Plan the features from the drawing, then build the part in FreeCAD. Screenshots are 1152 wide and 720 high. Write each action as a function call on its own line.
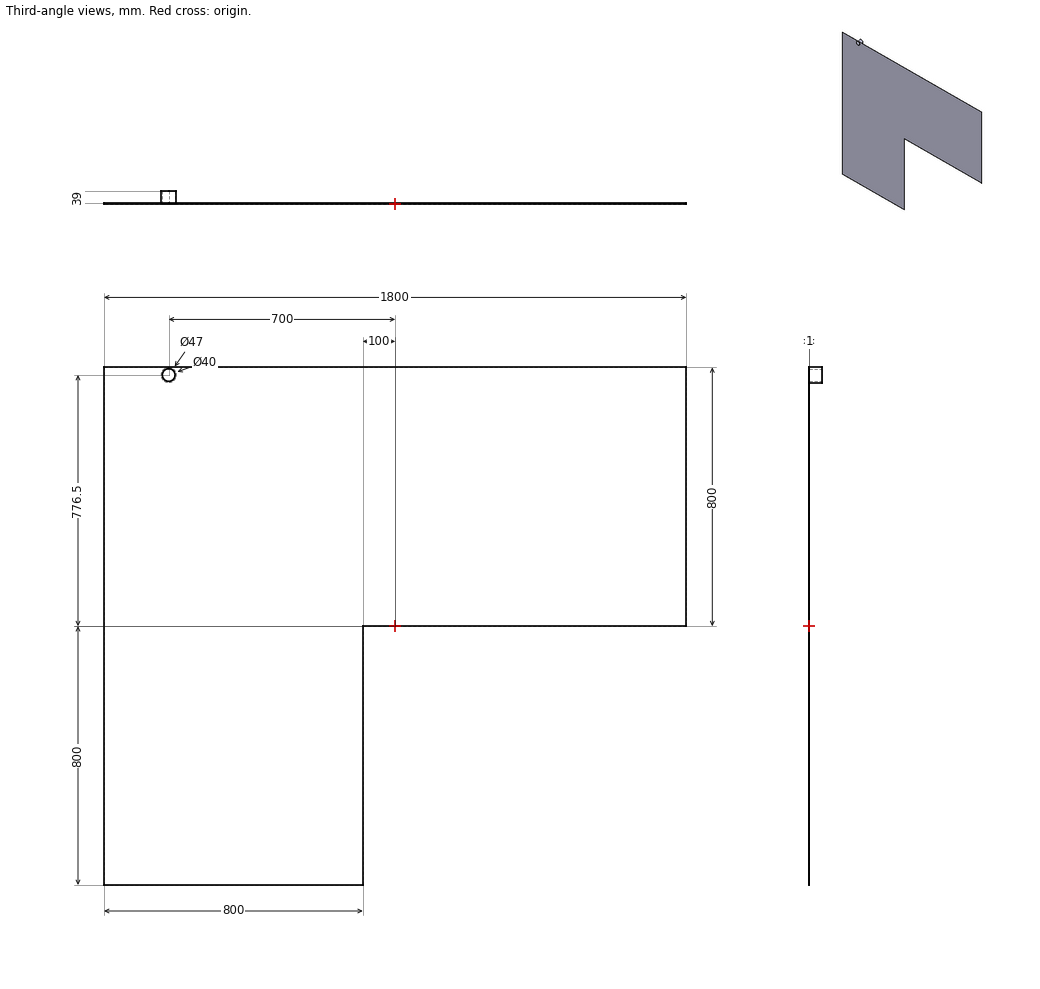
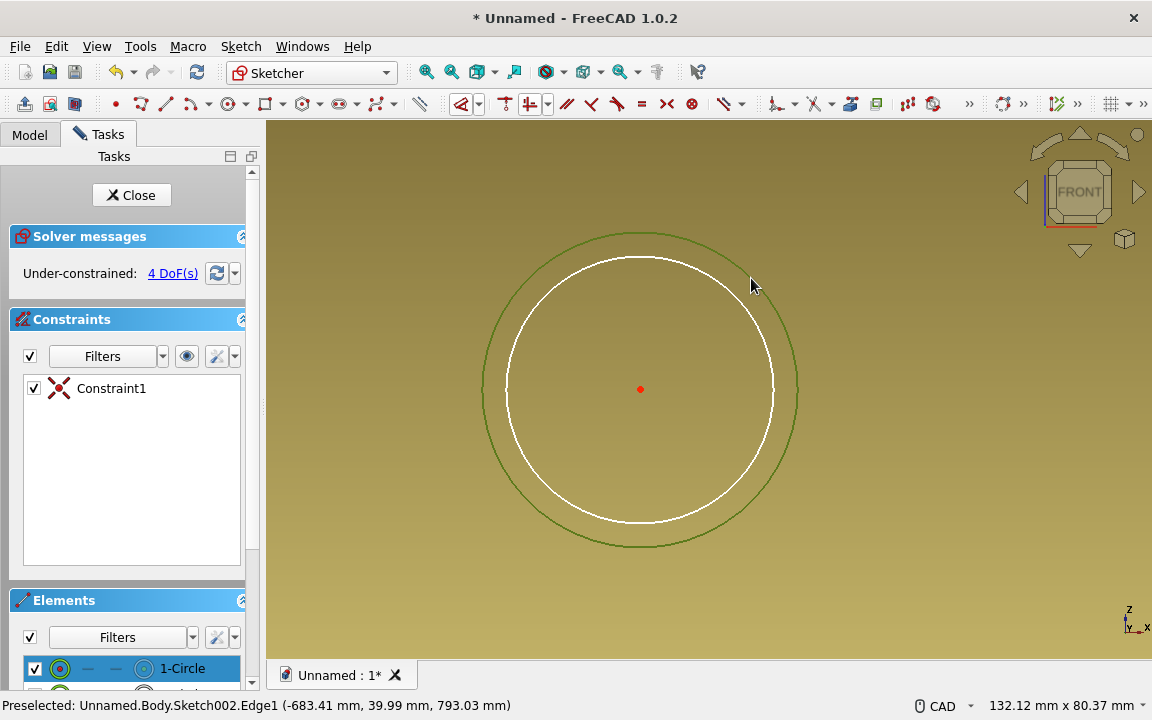
click(478, 104)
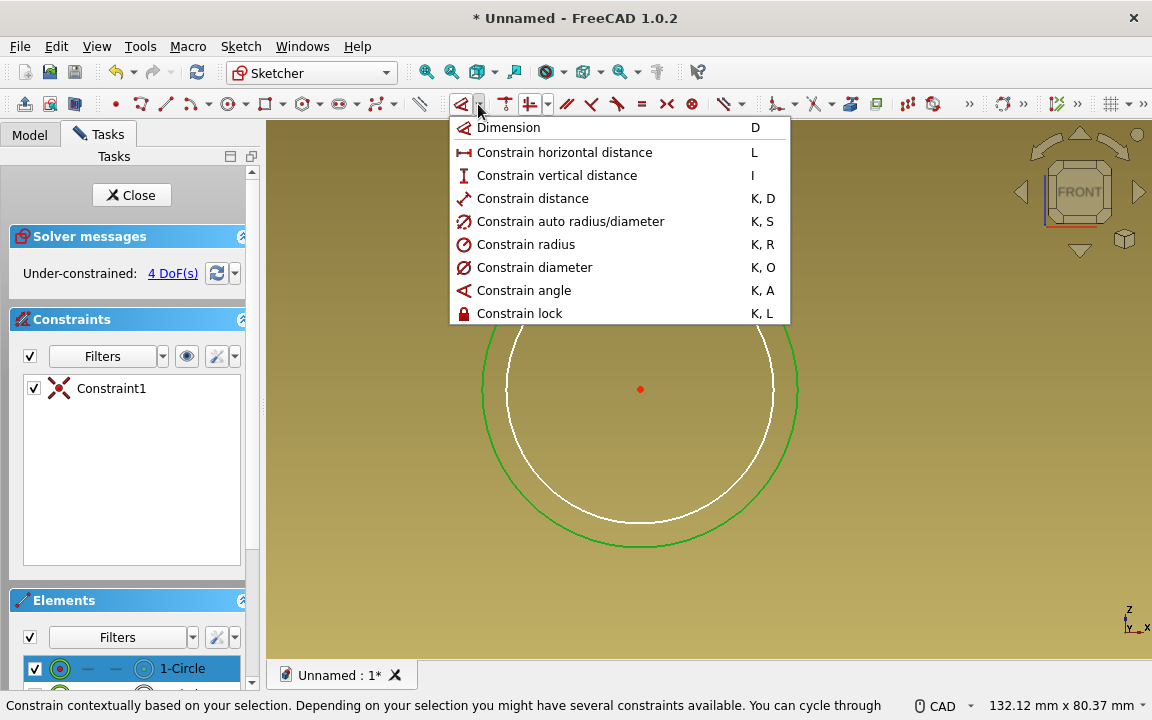
click(620, 268)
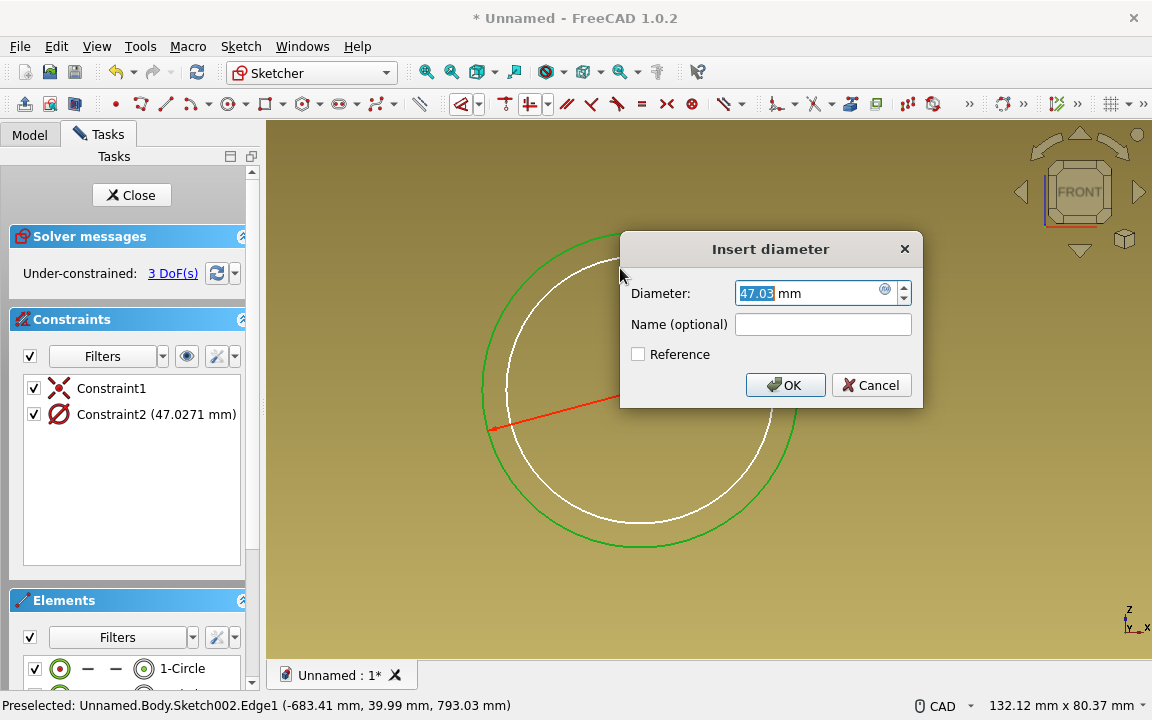
text(47)
key(Return)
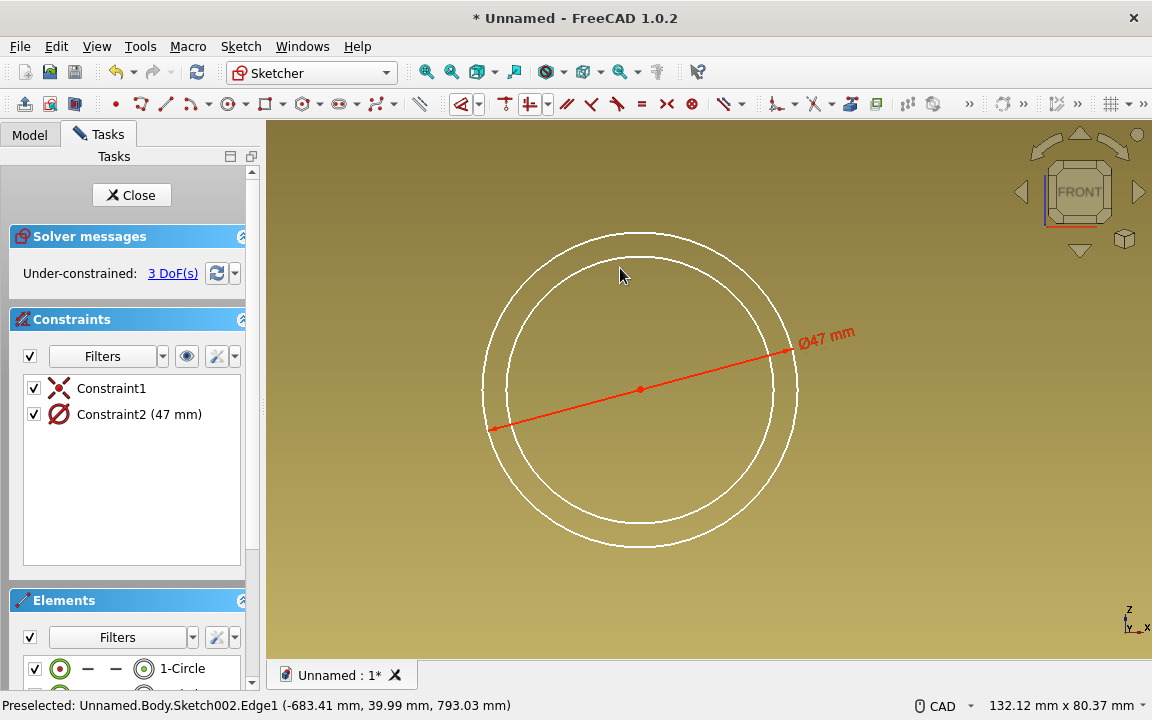
click(734, 295)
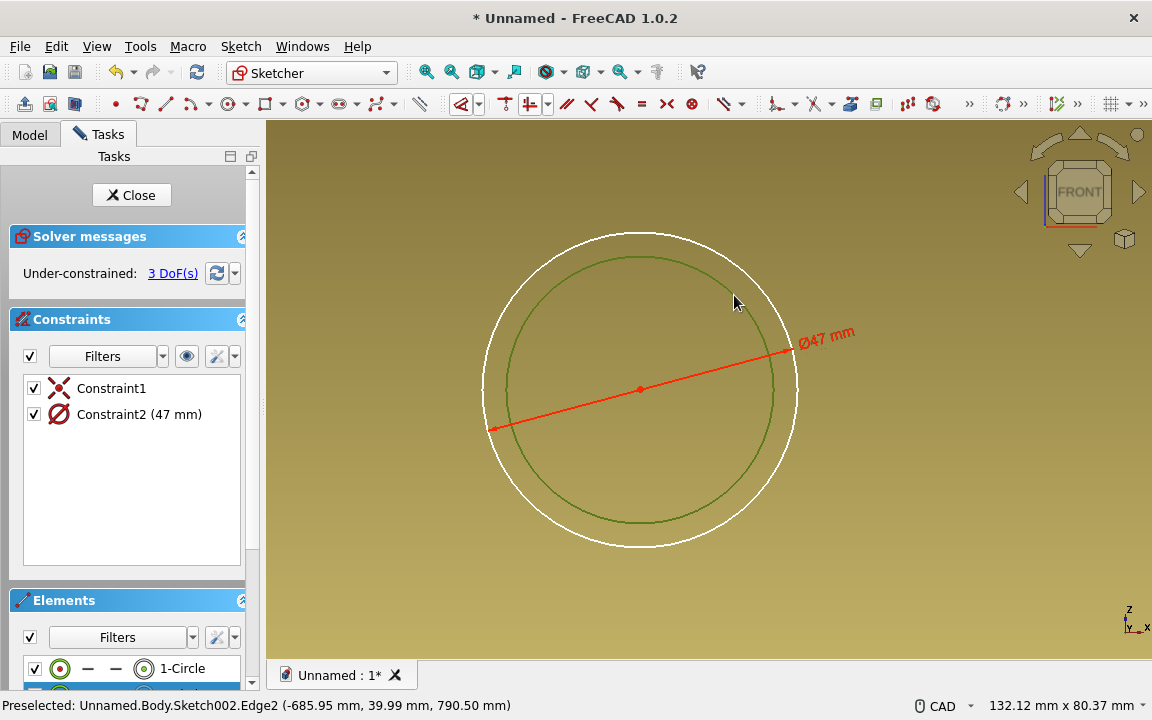
click(478, 104)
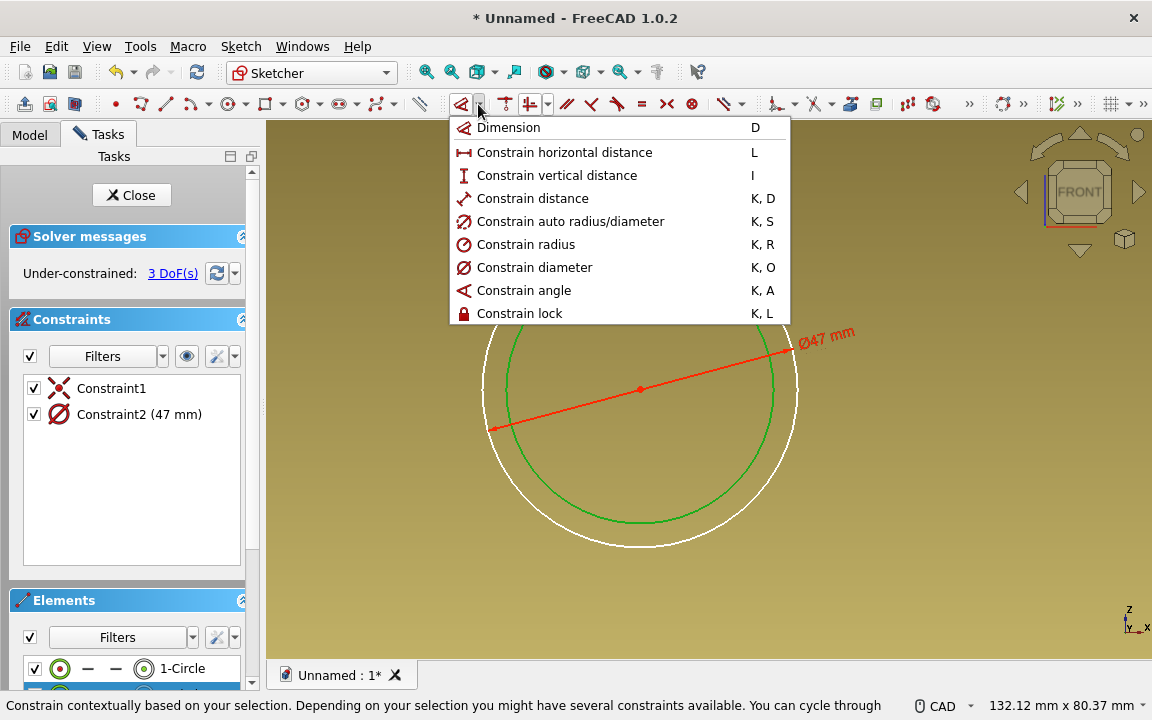
click(620, 268)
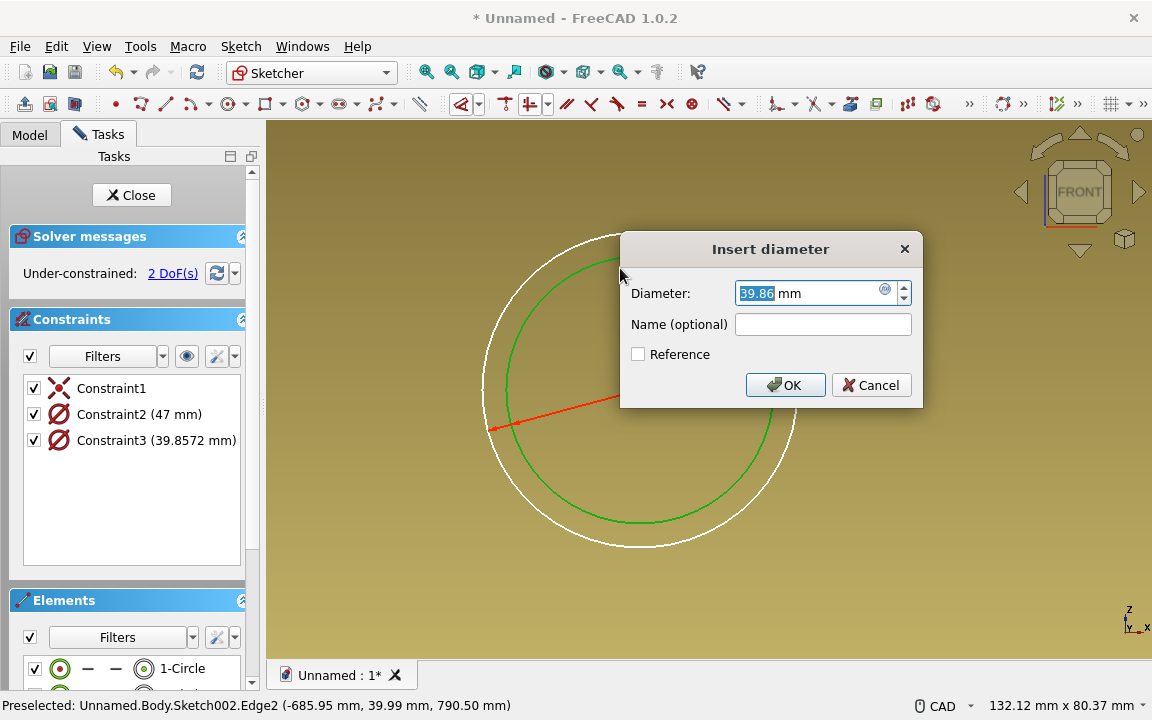
text(40)
key(Return)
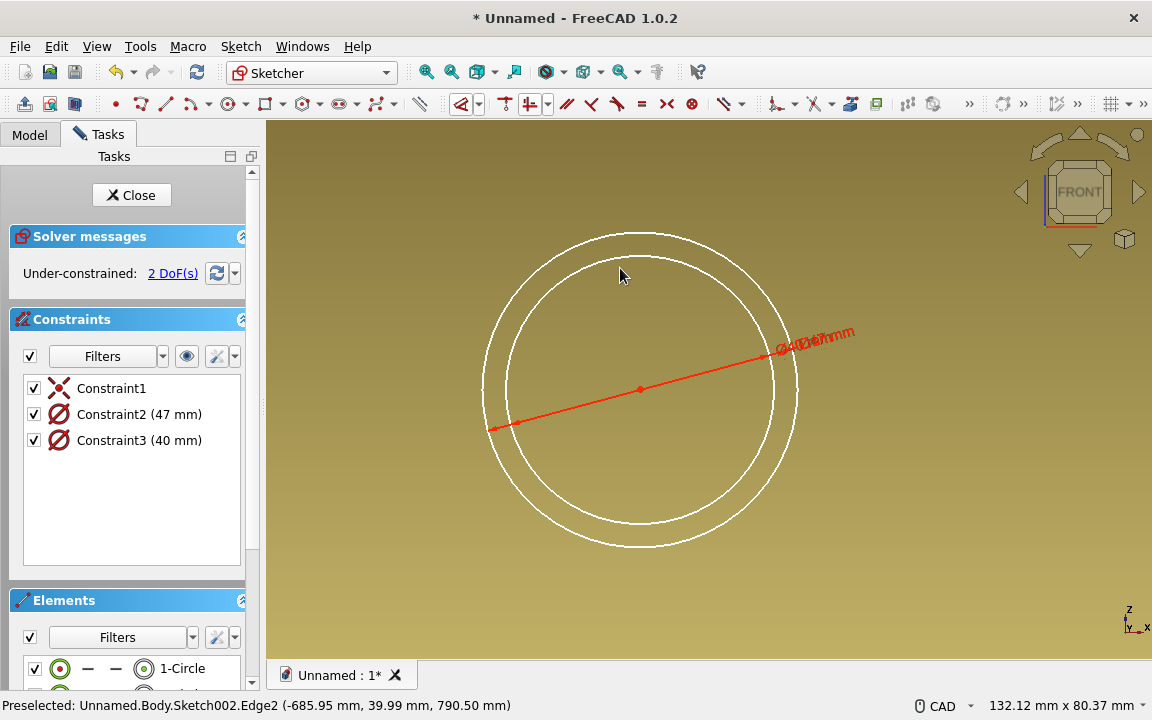
click(640, 390)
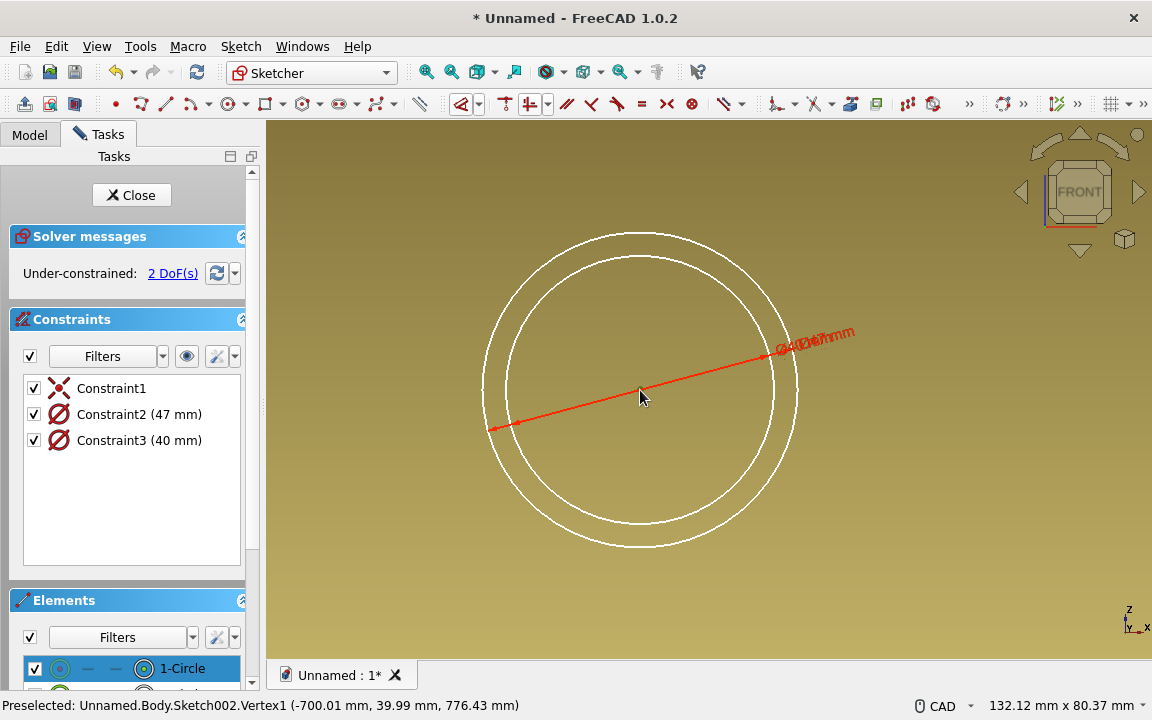
key(l)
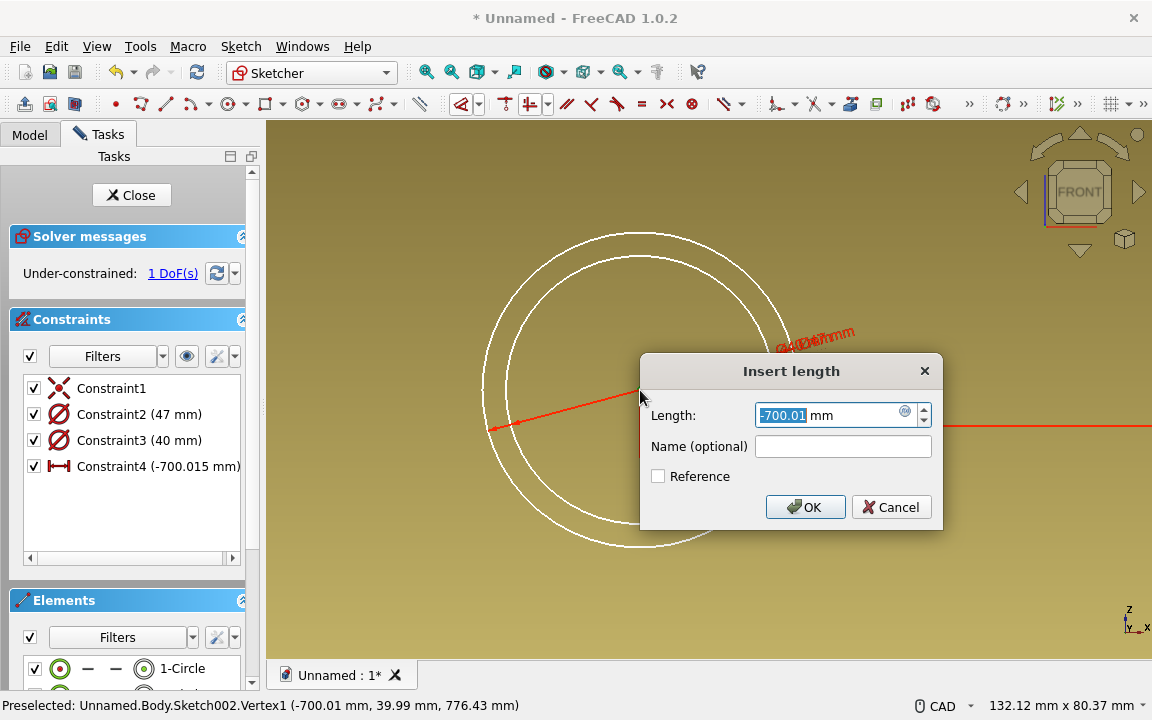
text(-700)
key(Return)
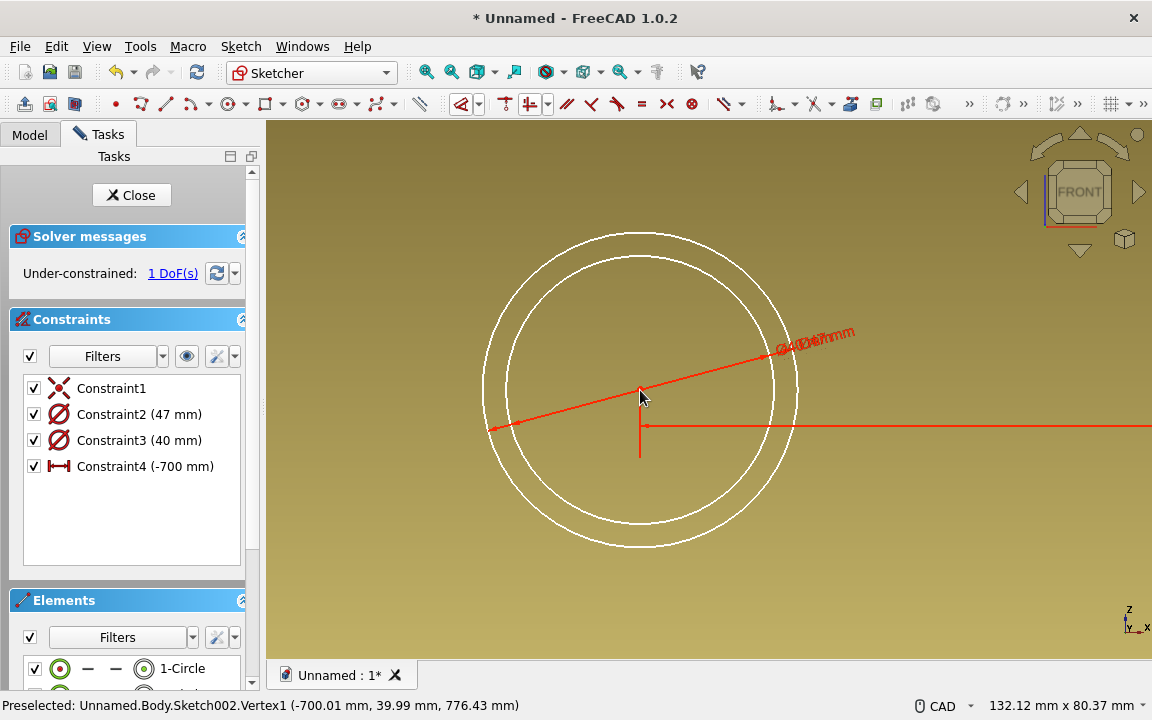
click(640, 390)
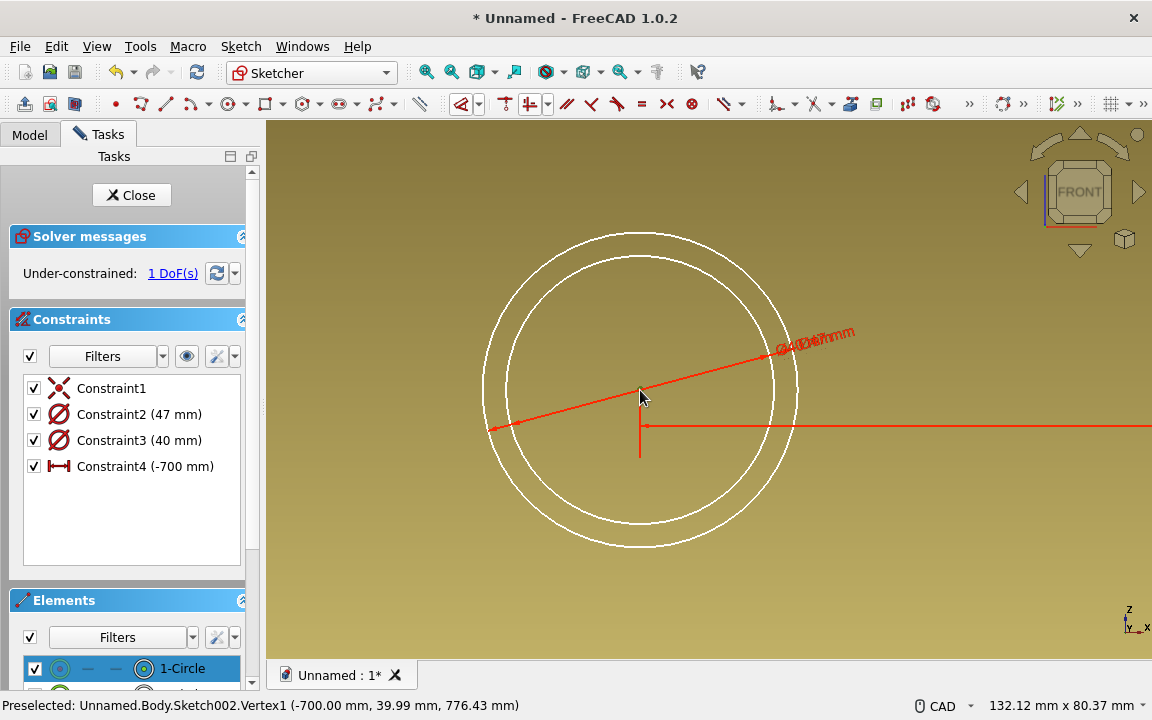
key(i)